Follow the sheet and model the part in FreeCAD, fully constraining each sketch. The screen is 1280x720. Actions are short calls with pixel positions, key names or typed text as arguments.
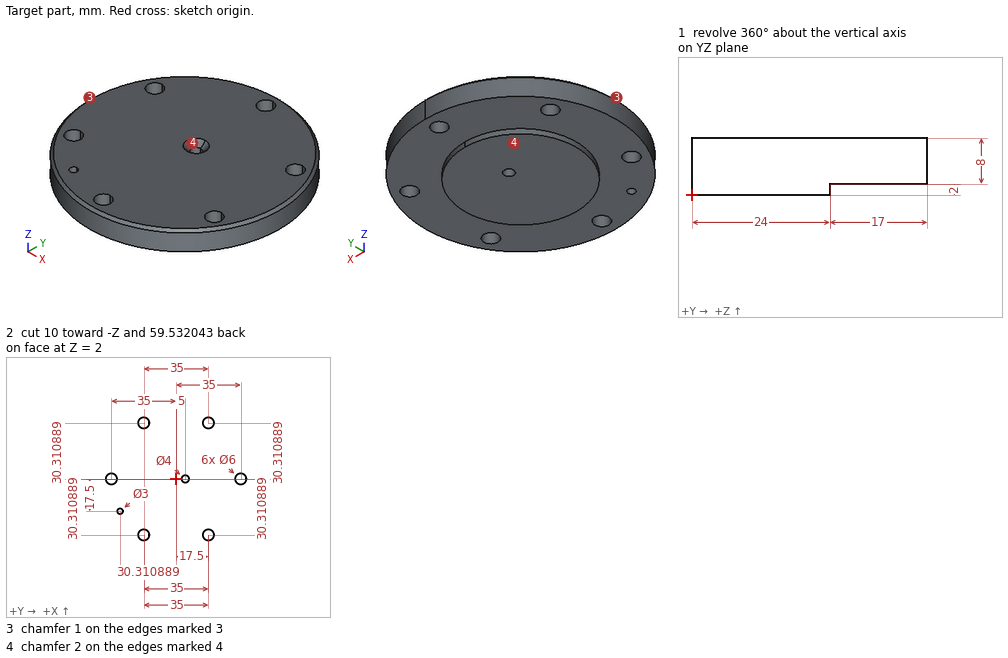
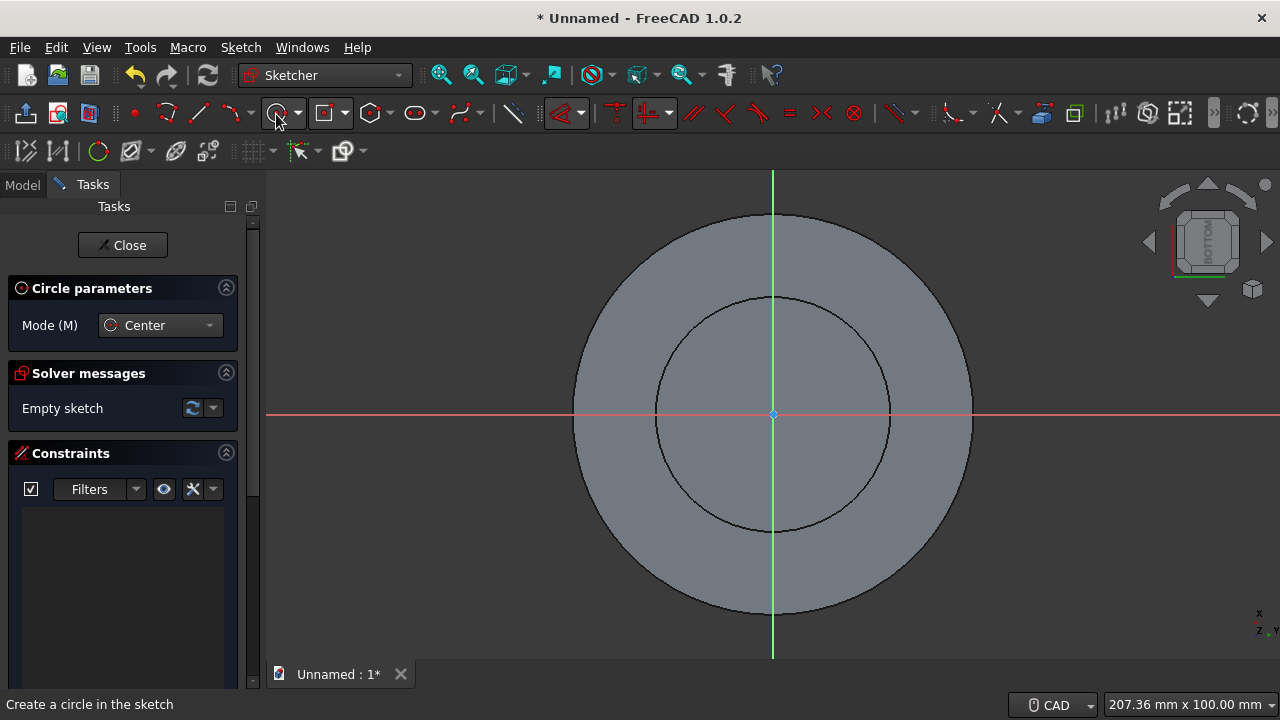
scroll(944, 415, up, 3)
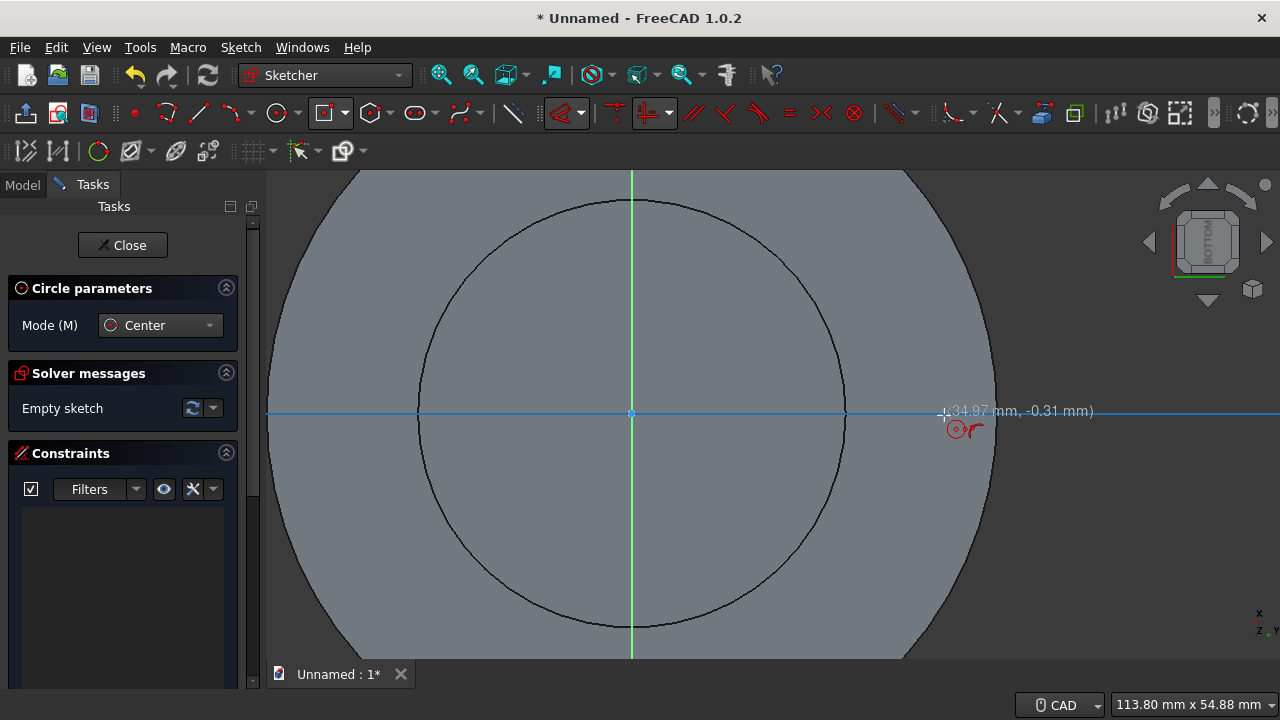
click(944, 414)
move(963, 395)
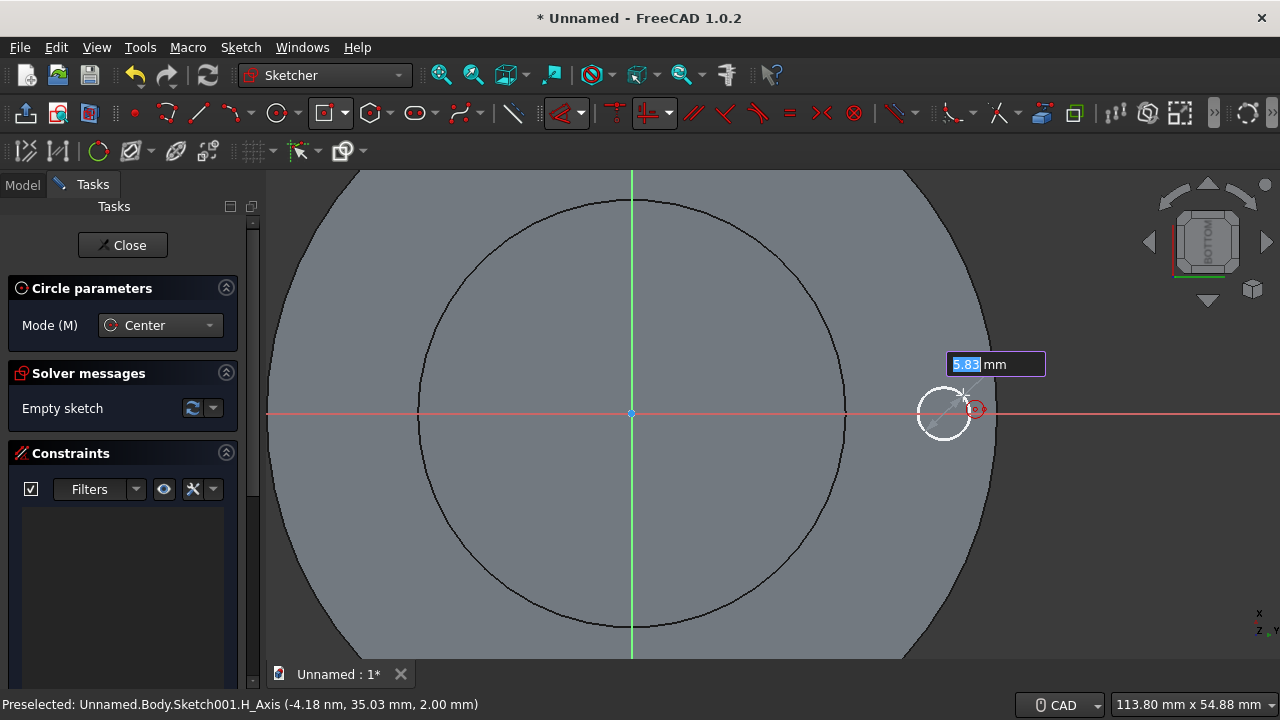
text(6)
key(Return)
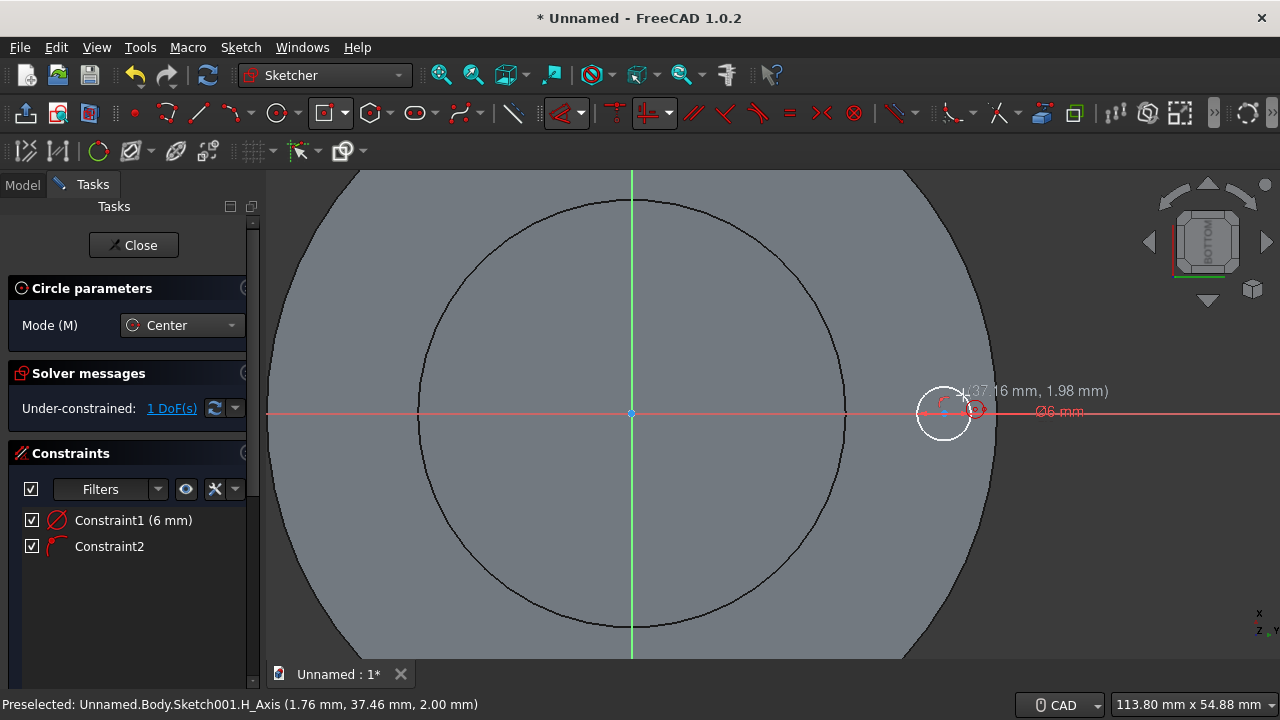
scroll(793, 416, down, 3)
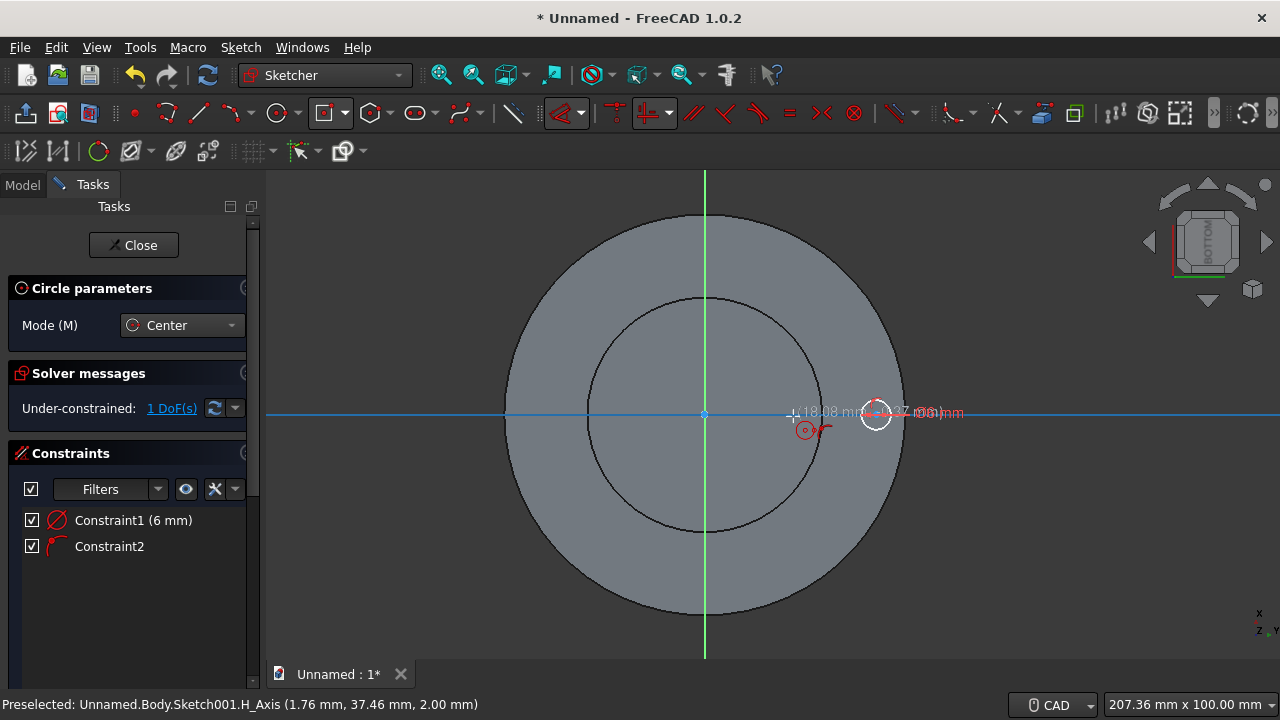
scroll(790, 563, up, 3)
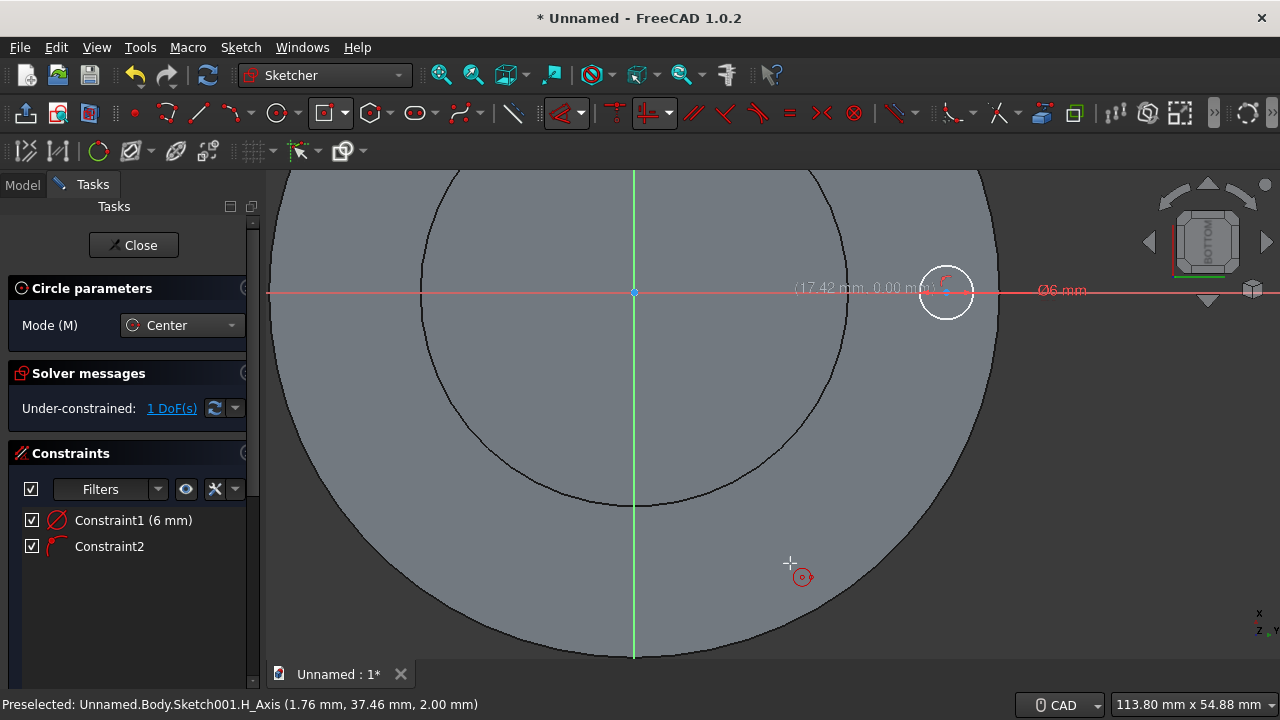
click(790, 563)
move(809, 544)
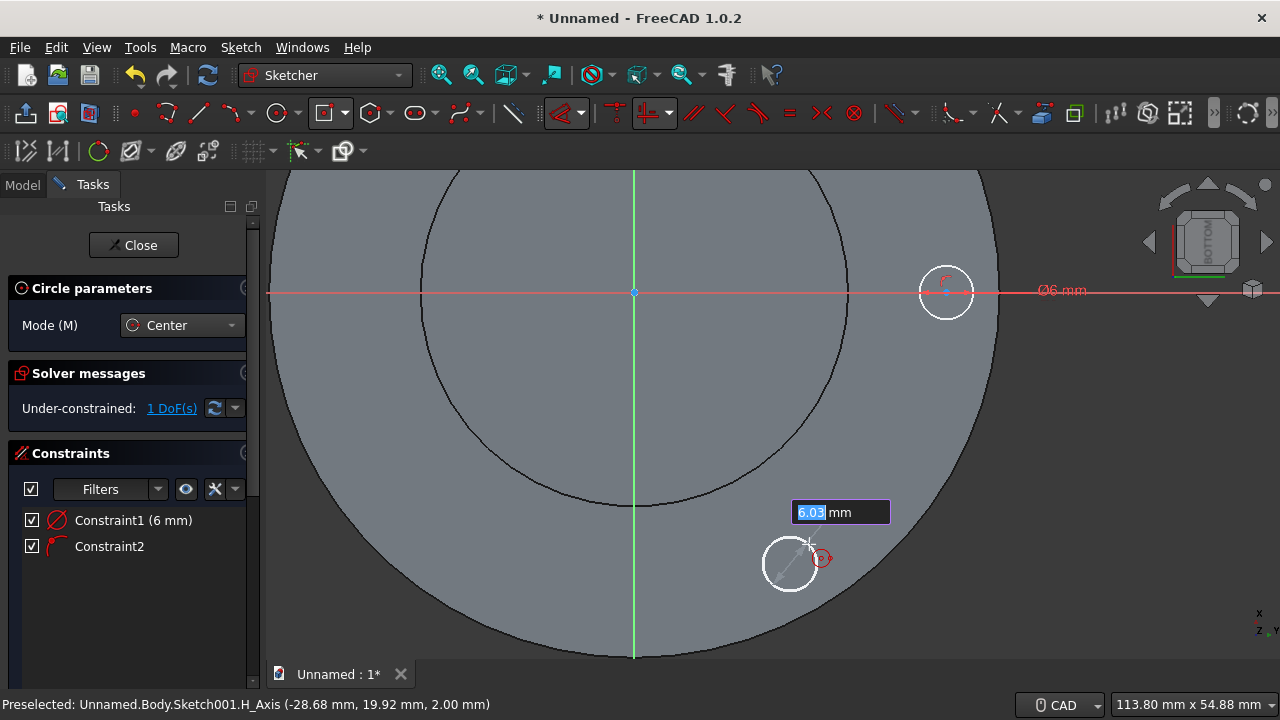
text(6)
key(Return)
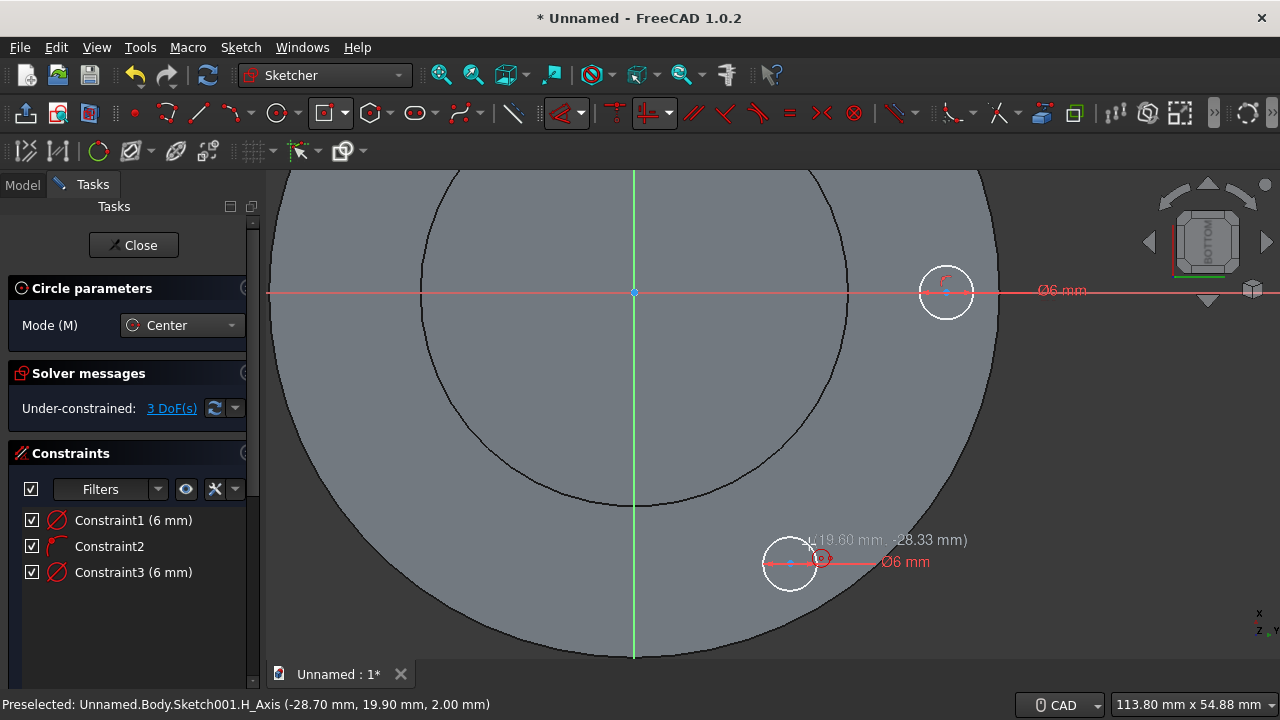
click(478, 563)
move(497, 544)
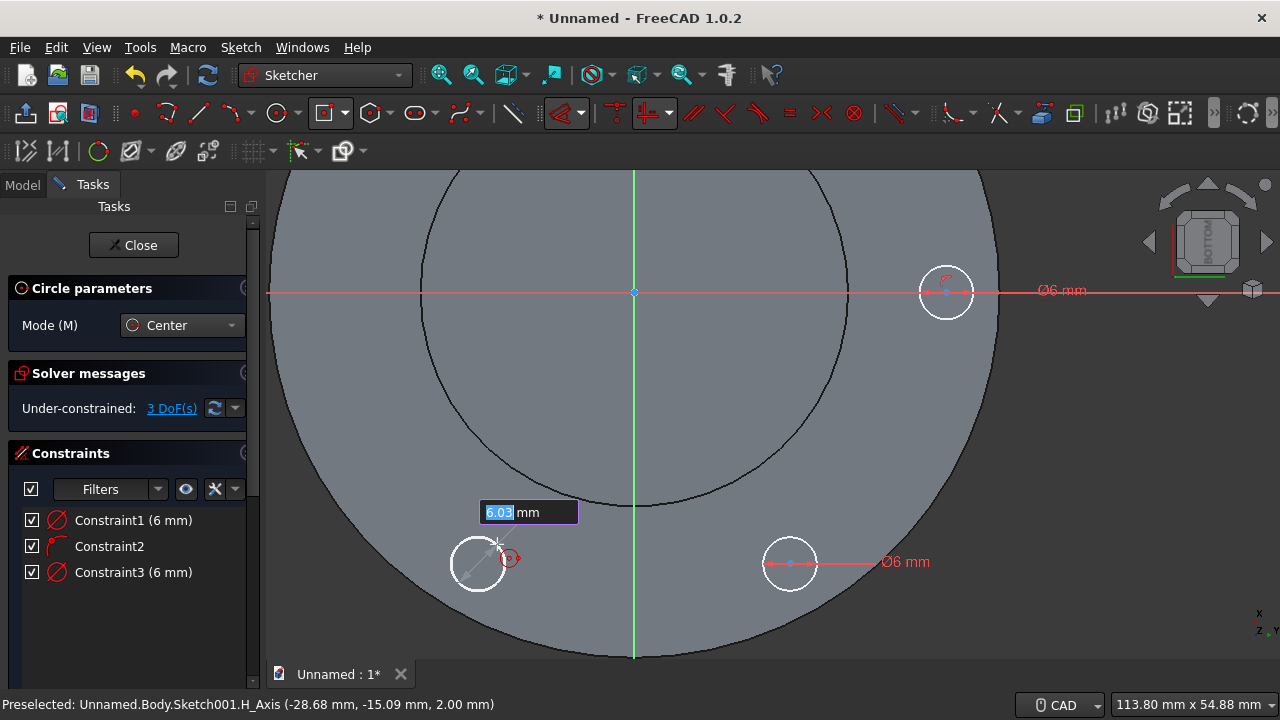
text(6)
key(Return)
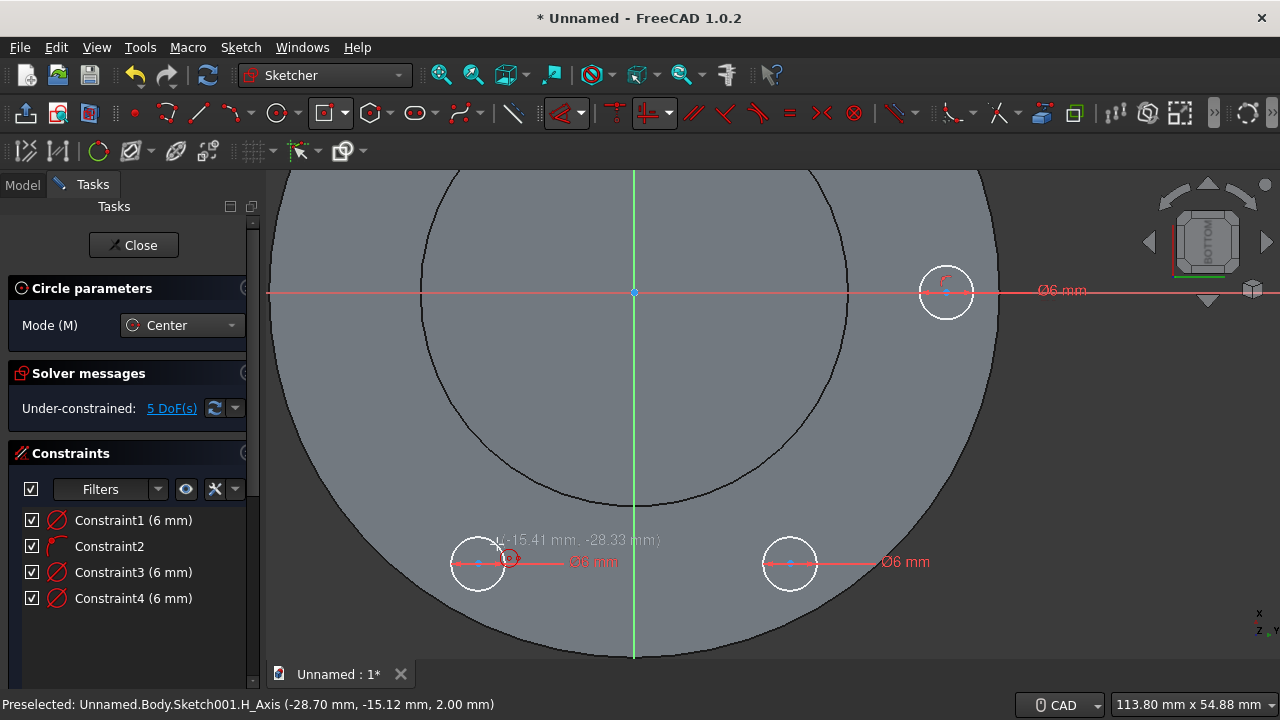
click(322, 293)
move(341, 274)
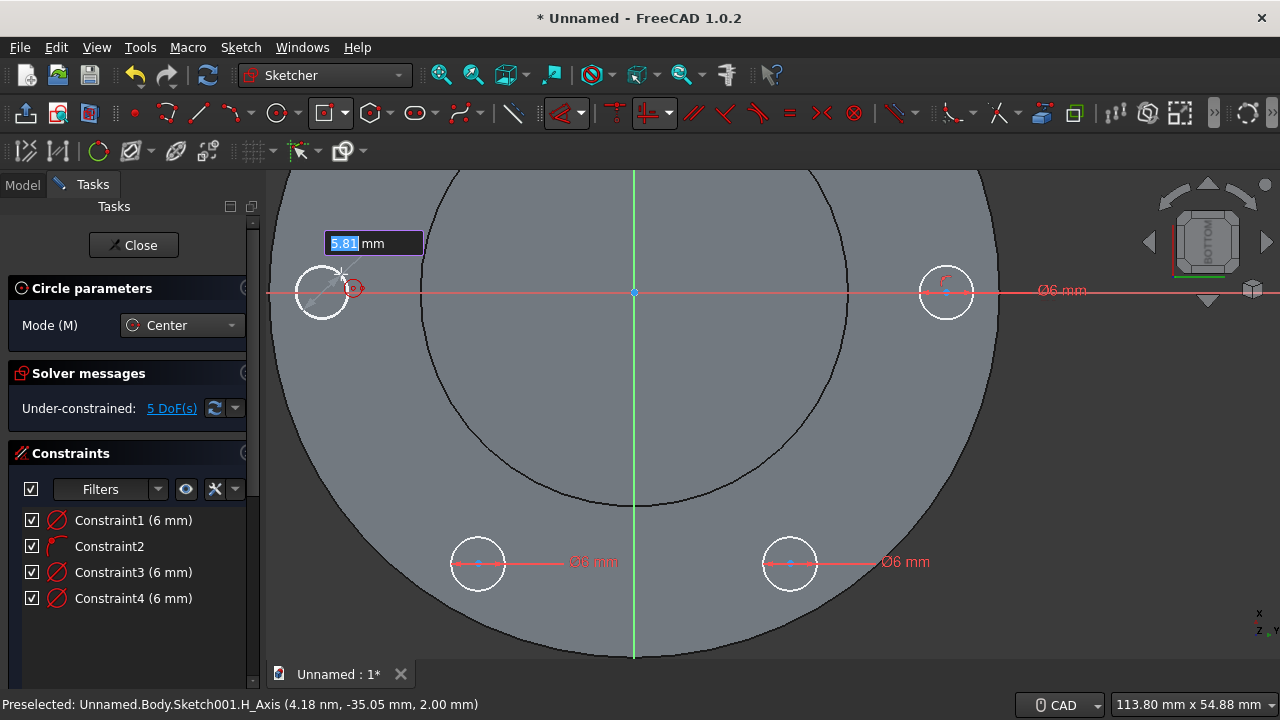
text(6)
key(Return)